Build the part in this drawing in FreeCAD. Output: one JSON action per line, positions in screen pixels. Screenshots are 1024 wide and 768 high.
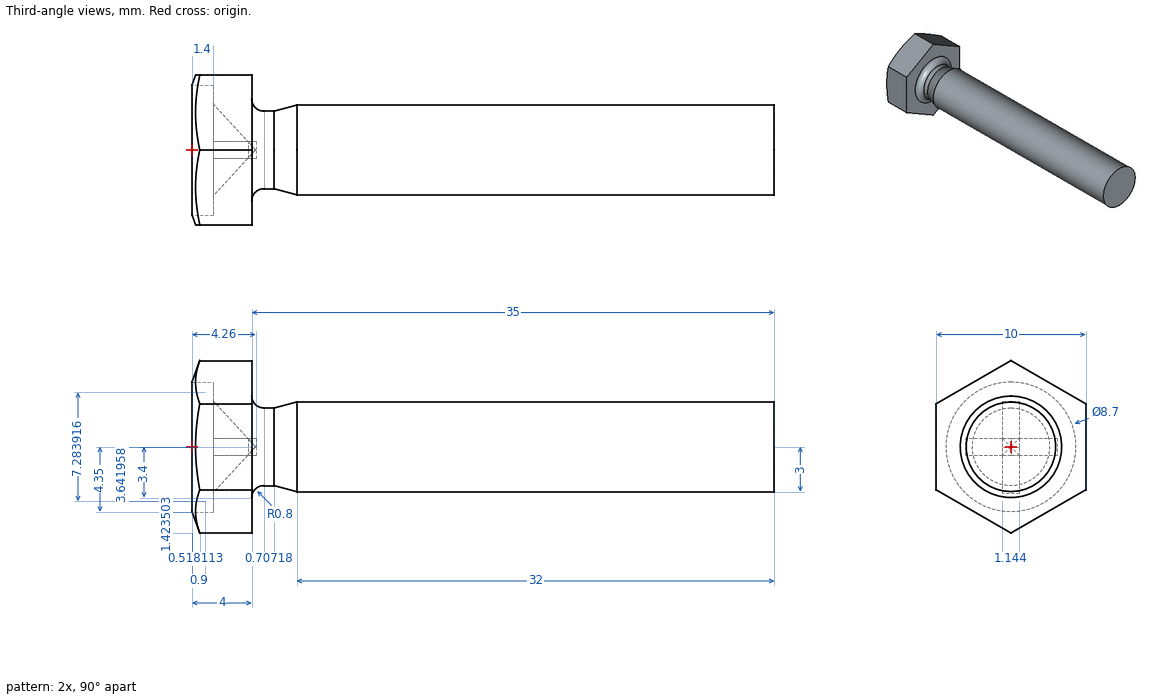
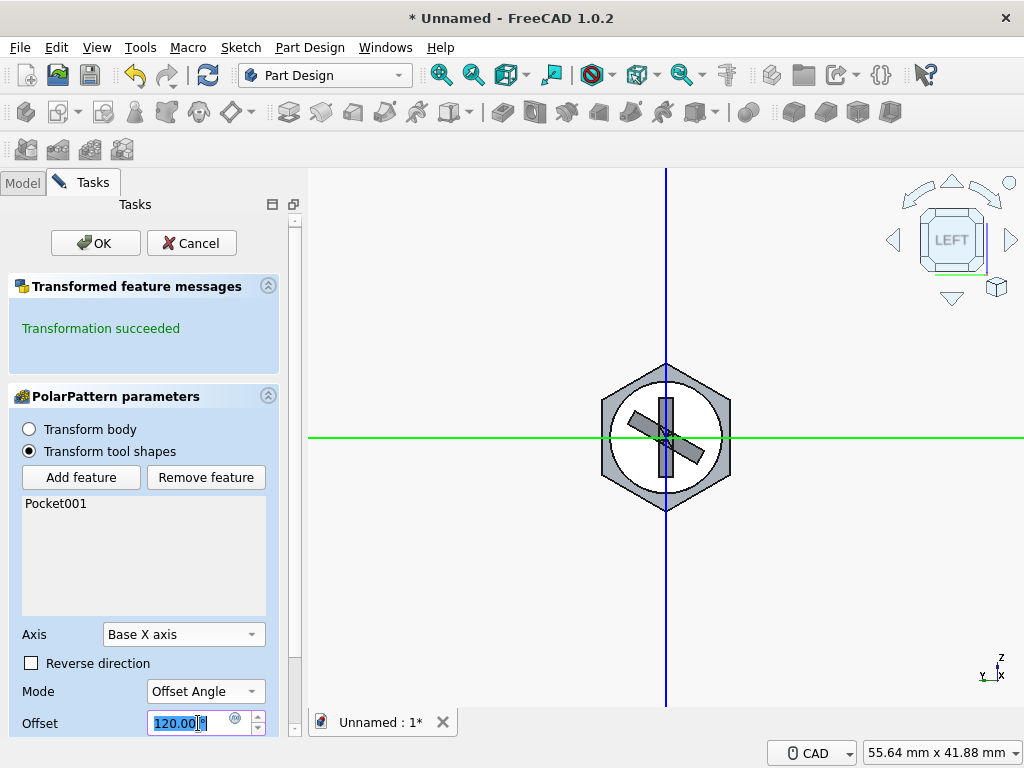
{"action": "type", "text": "90"}
{"action": "key", "text": "Tab"}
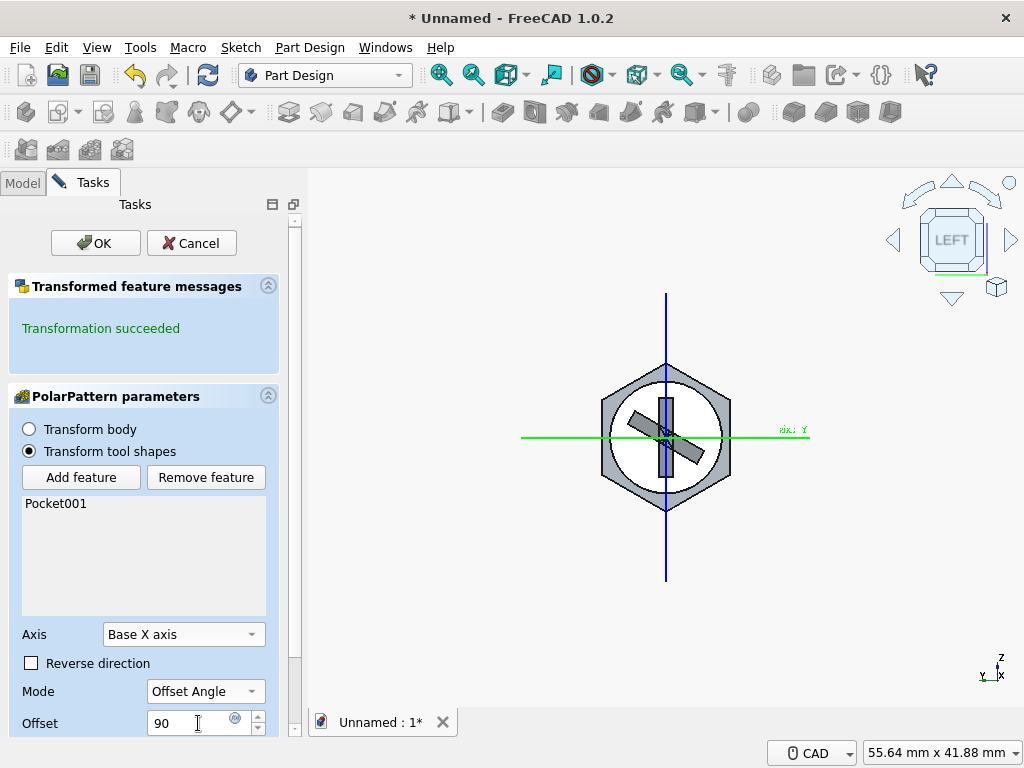
{"action": "scroll", "coordinate": [295, 475], "scroll_direction": "down", "scroll_amount": 2}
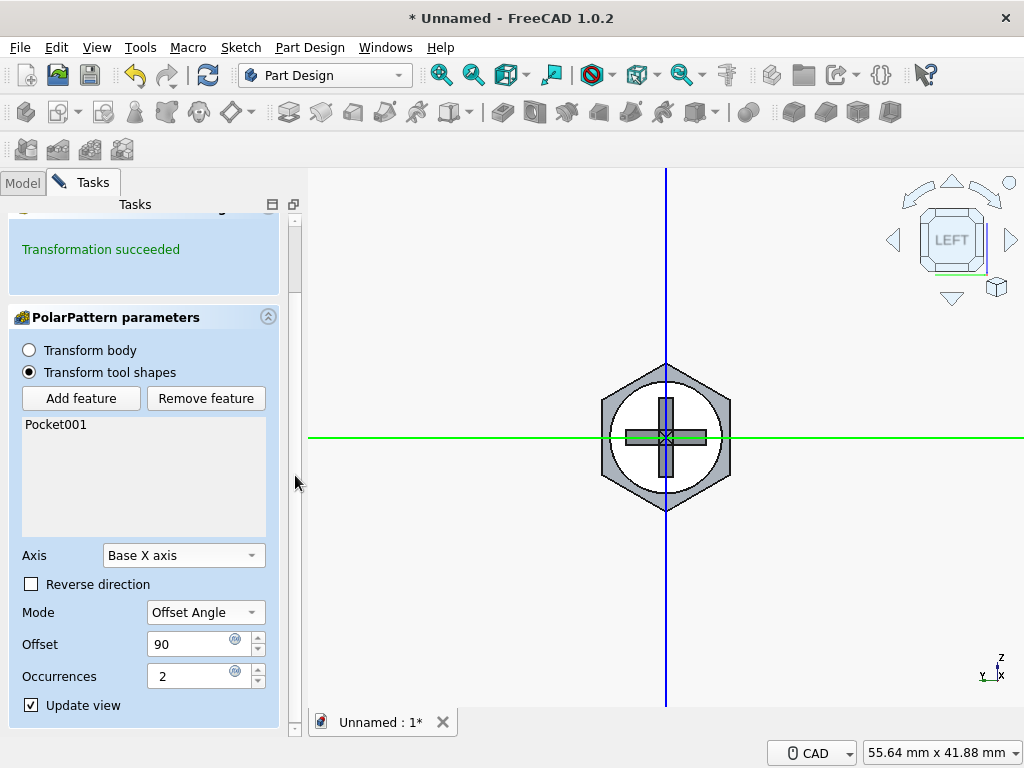
{"action": "triple_click", "coordinate": [198, 676]}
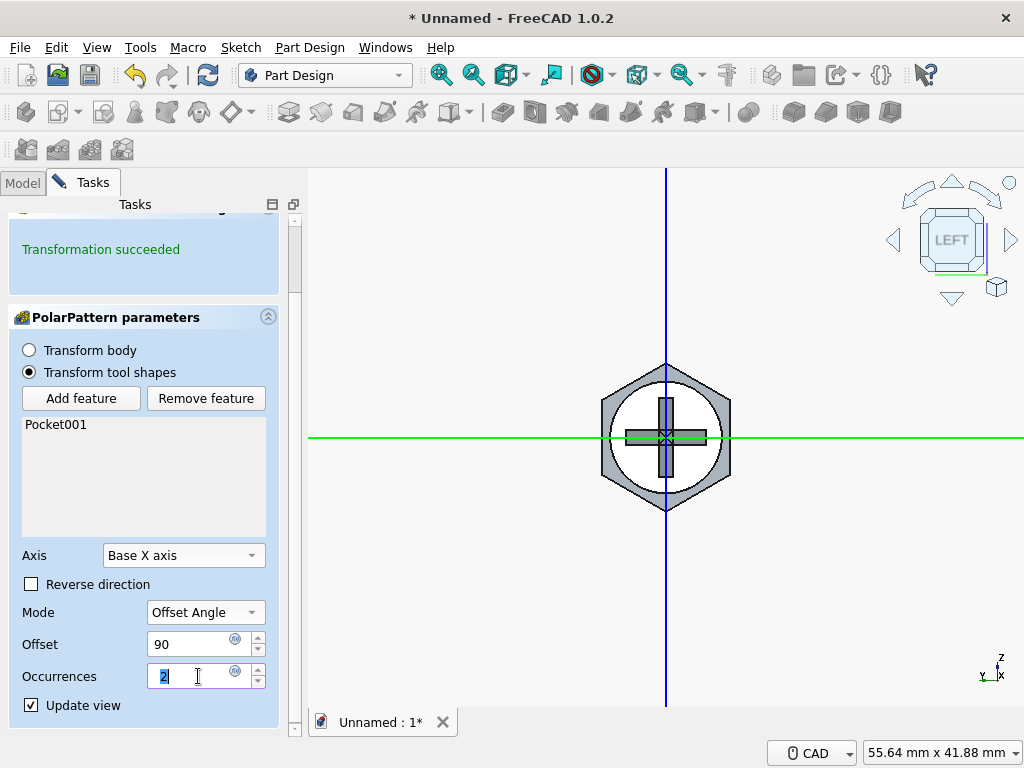
{"action": "type", "text": "2"}
{"action": "key", "text": "Tab"}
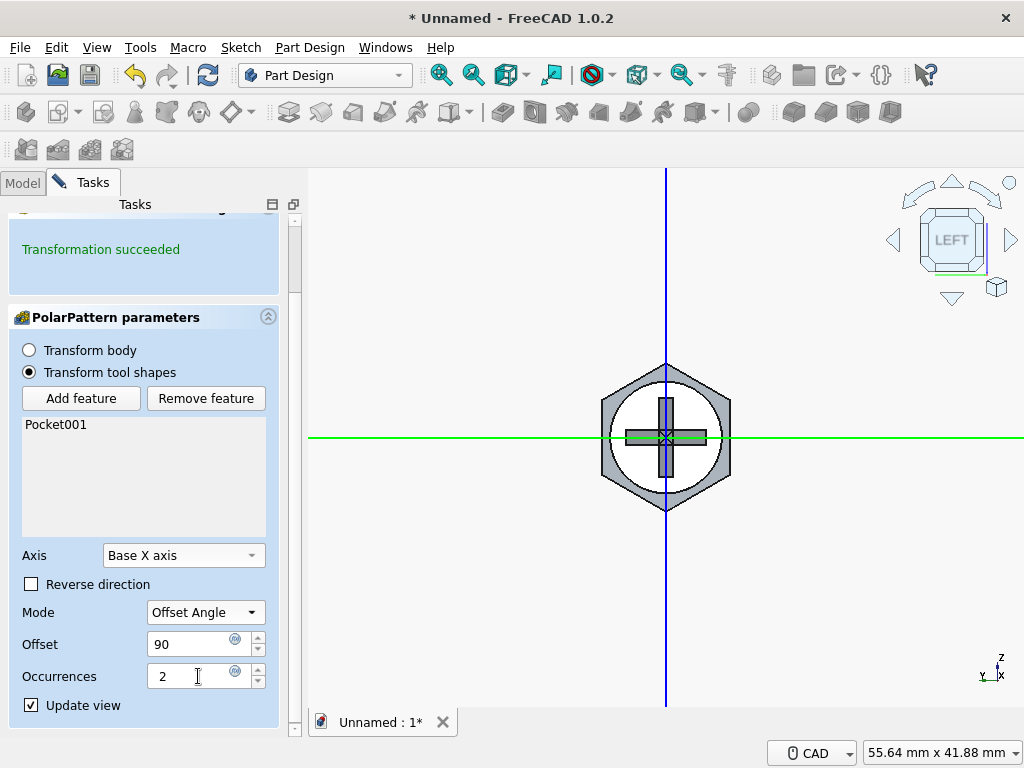
{"action": "scroll", "coordinate": [295, 475], "scroll_direction": "up", "scroll_amount": 3}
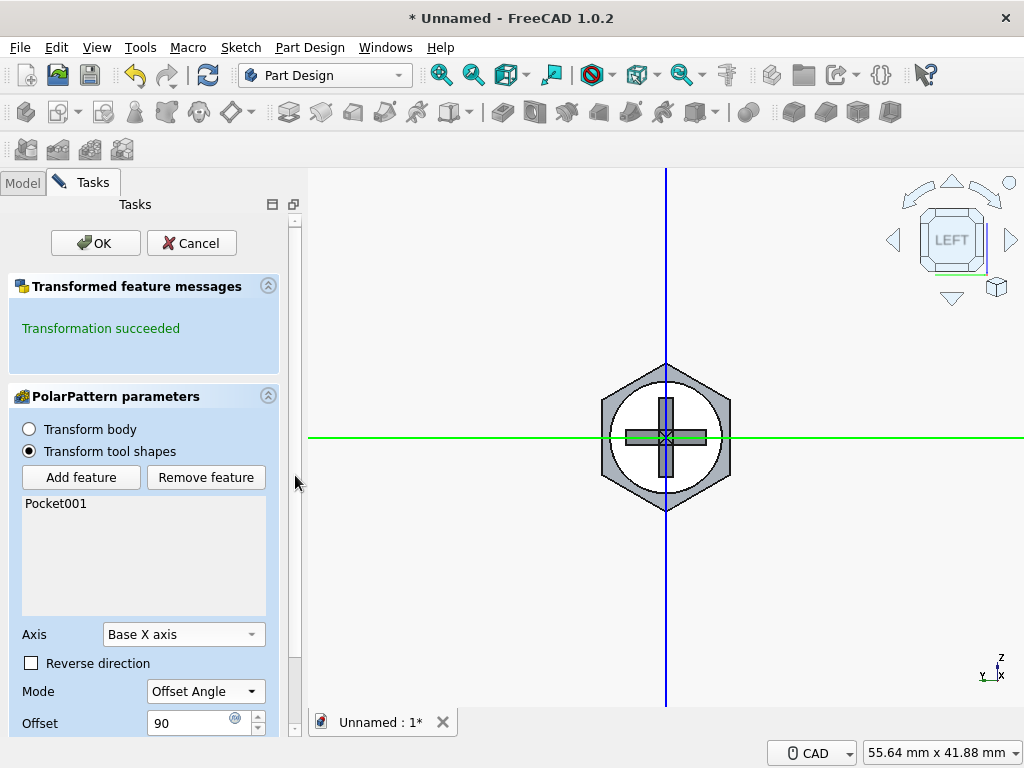
{"action": "left_click", "coordinate": [96, 243]}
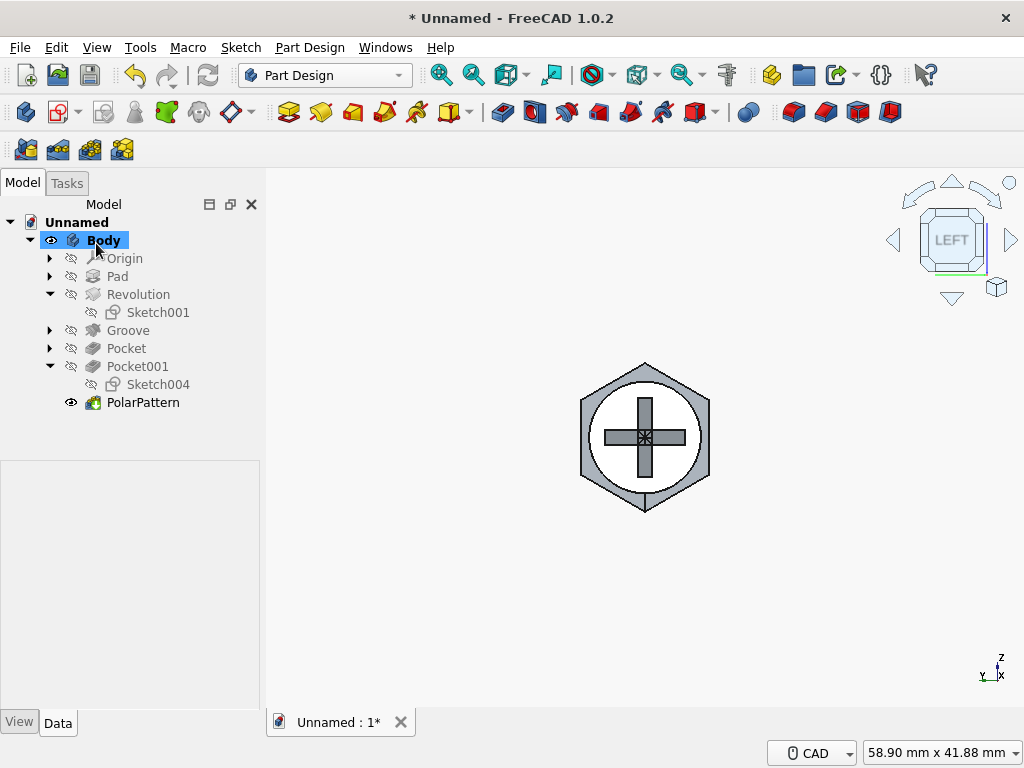
{"action": "key", "text": "0"}